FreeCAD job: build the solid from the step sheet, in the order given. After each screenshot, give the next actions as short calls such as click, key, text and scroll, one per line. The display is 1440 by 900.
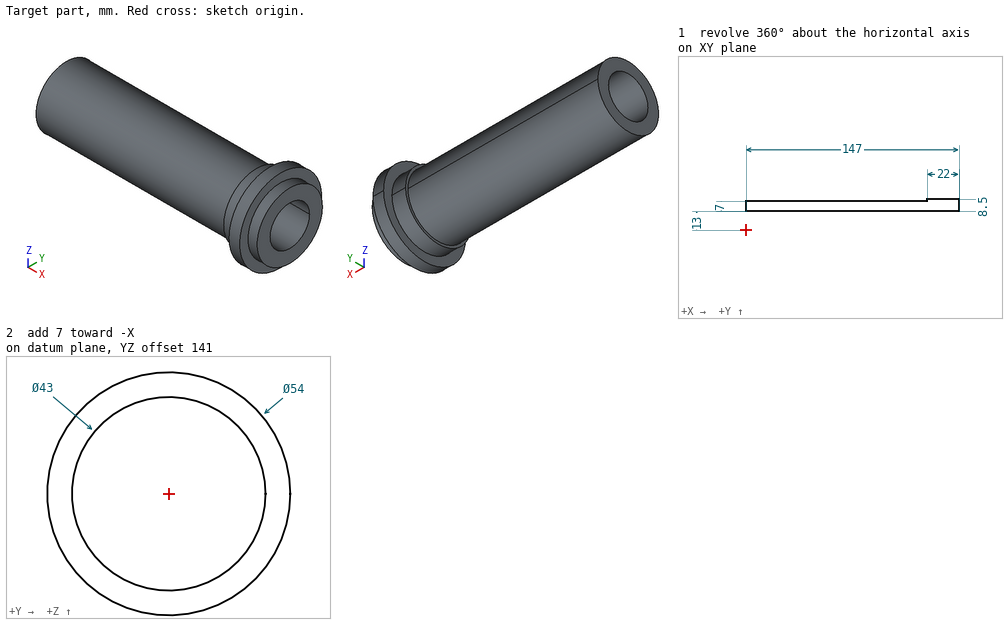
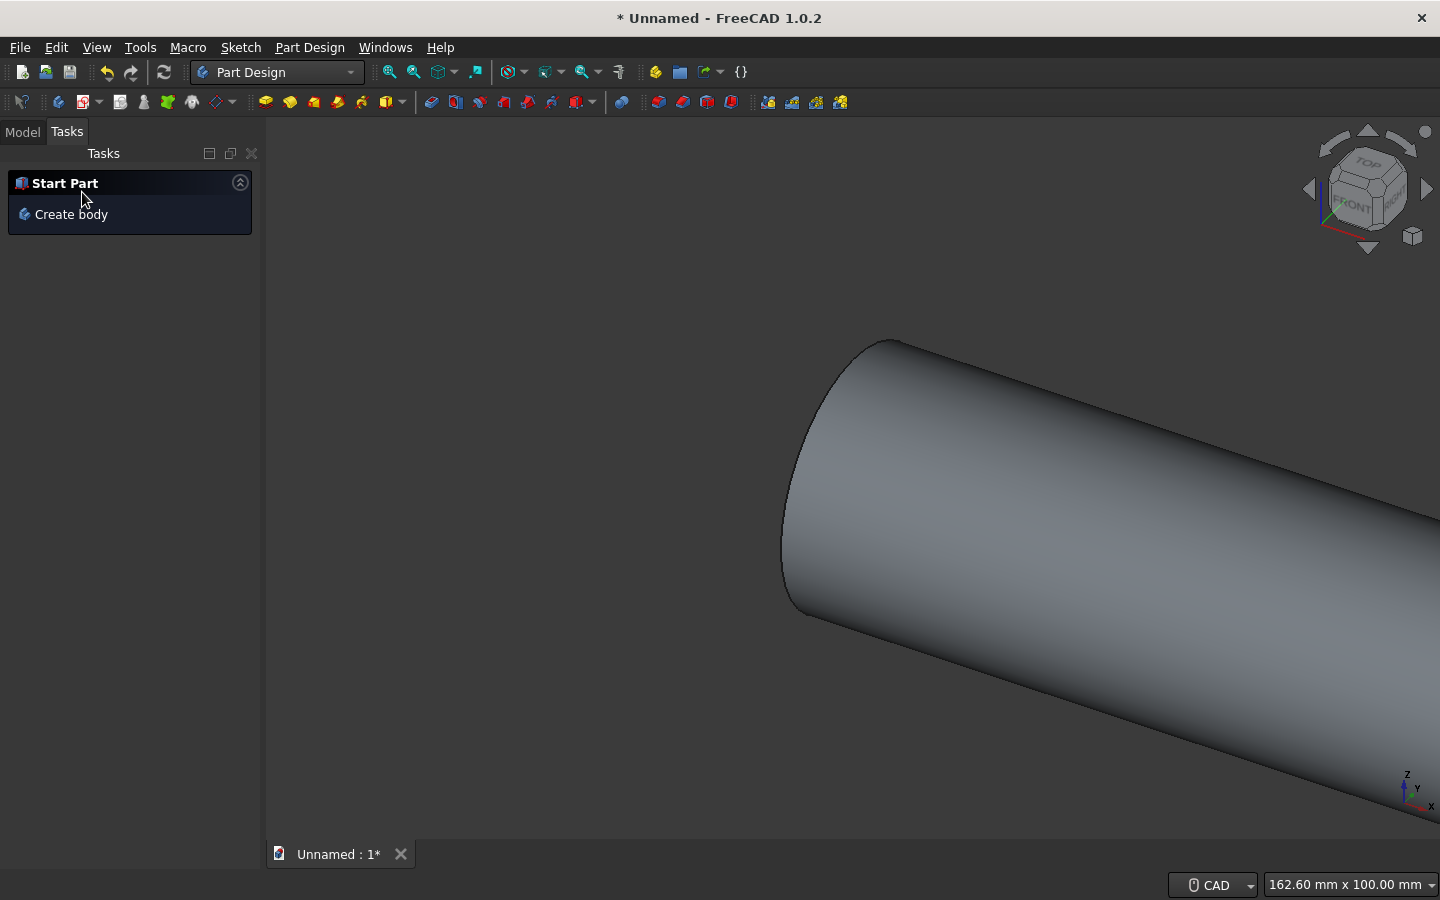
click(390, 72)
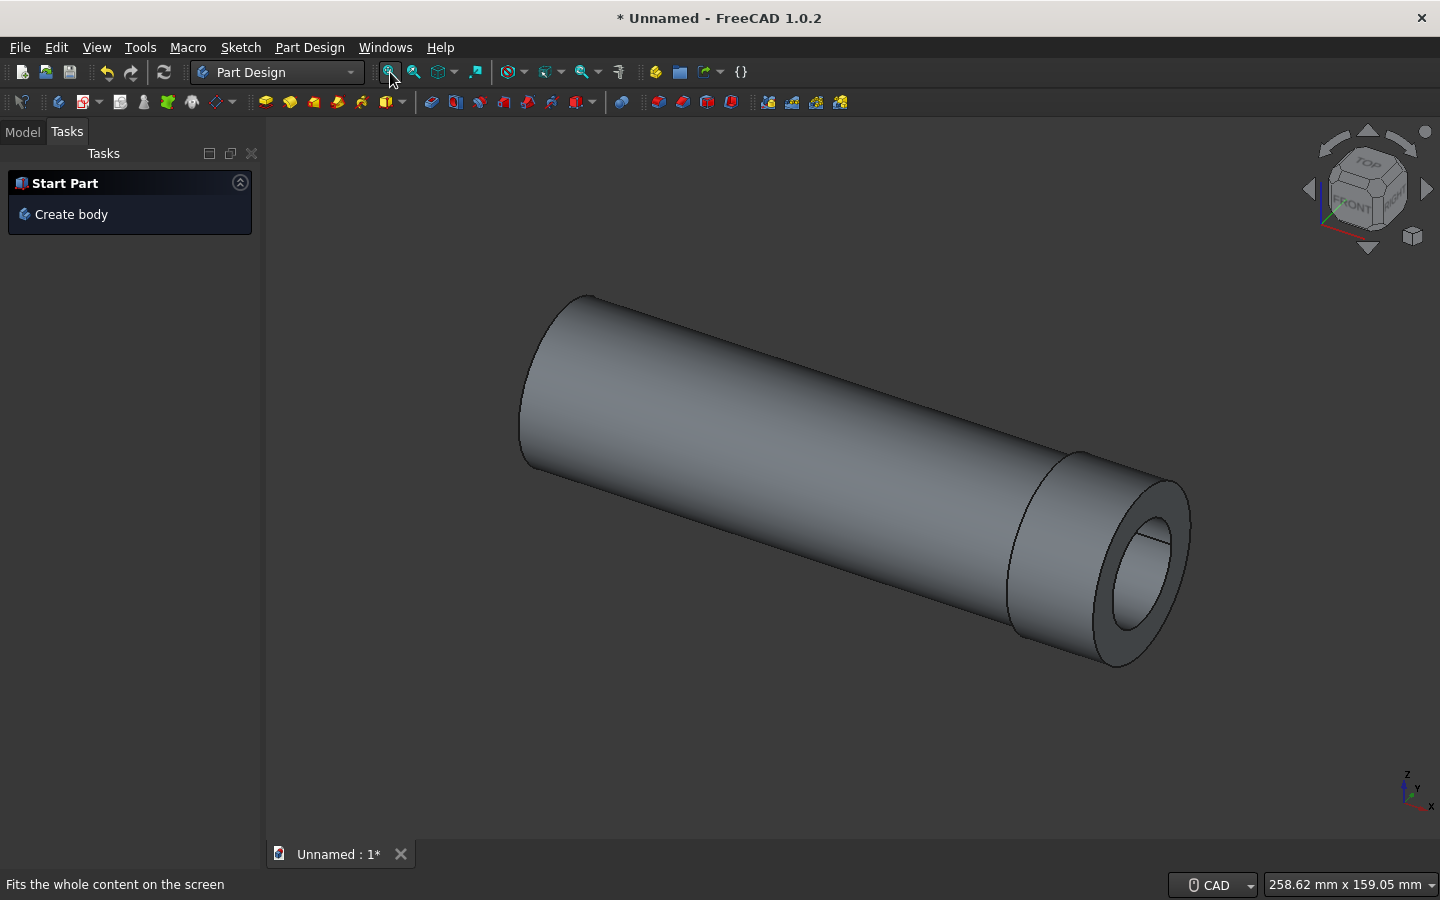
click(23, 131)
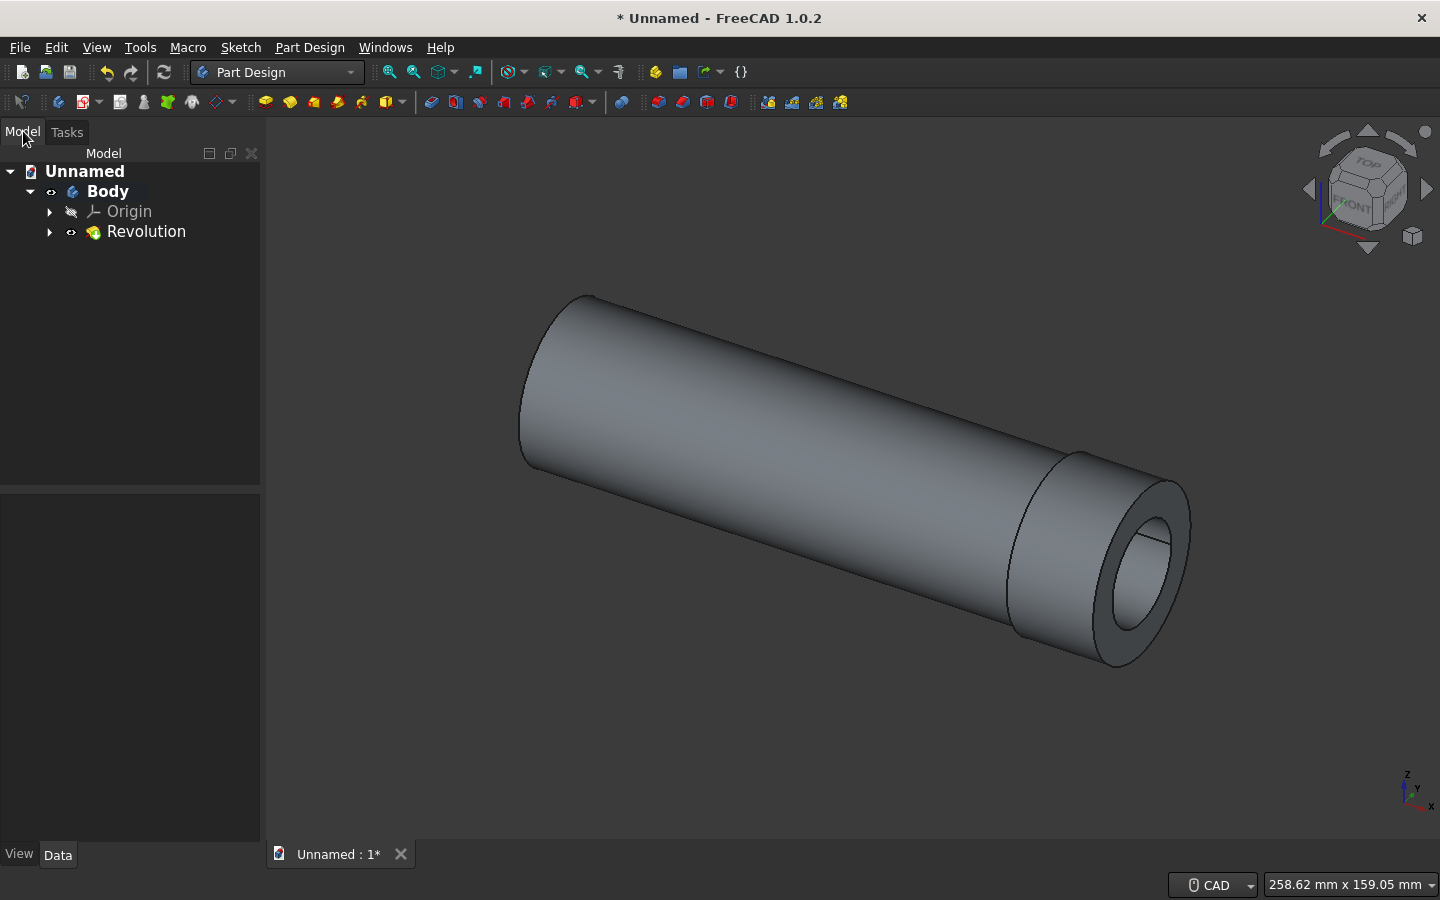
click(50, 212)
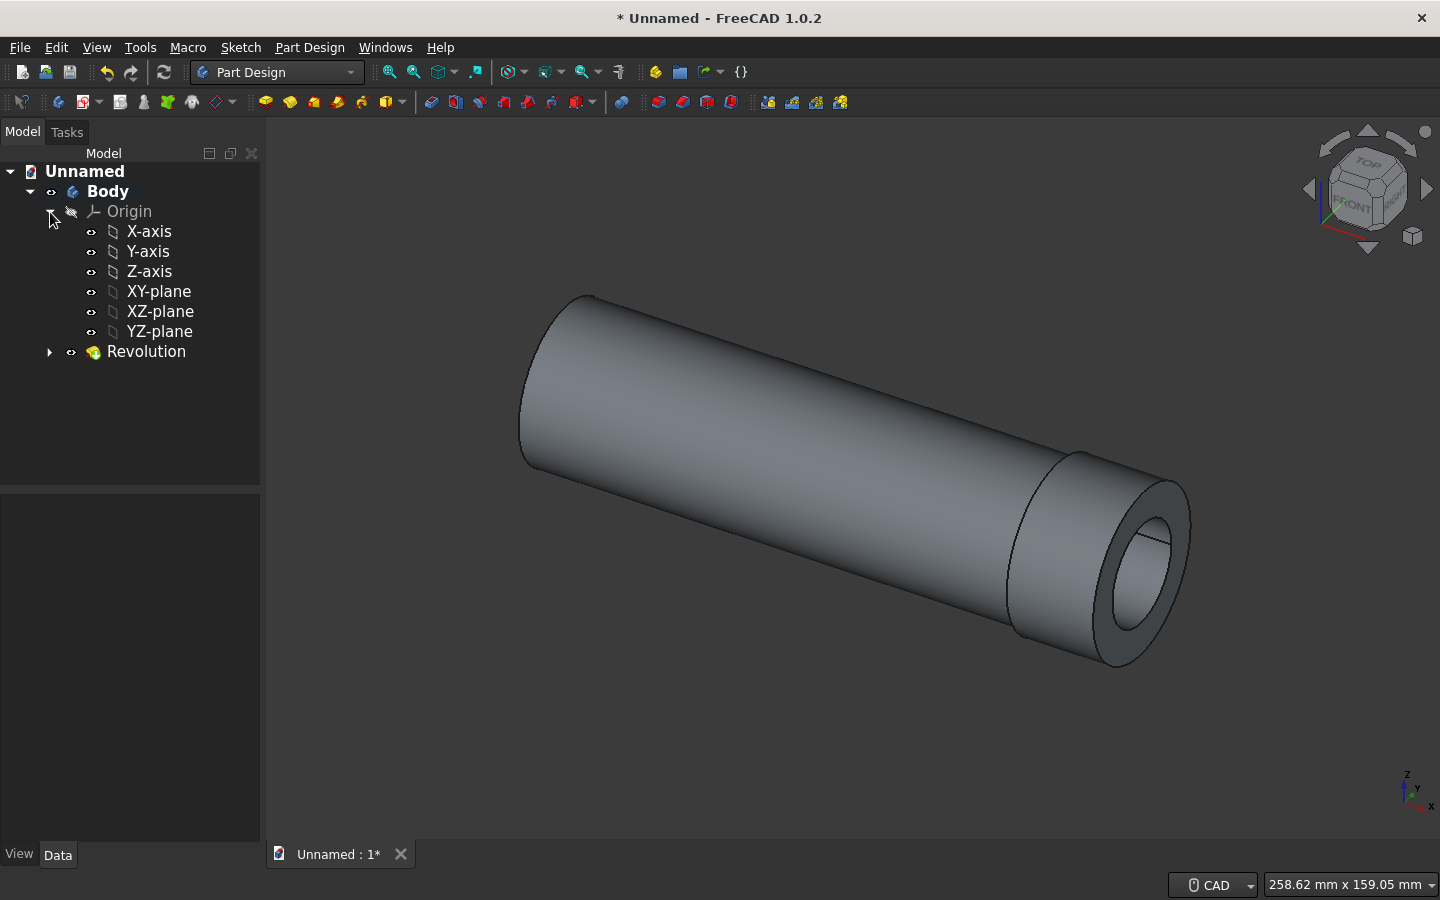
click(136, 332)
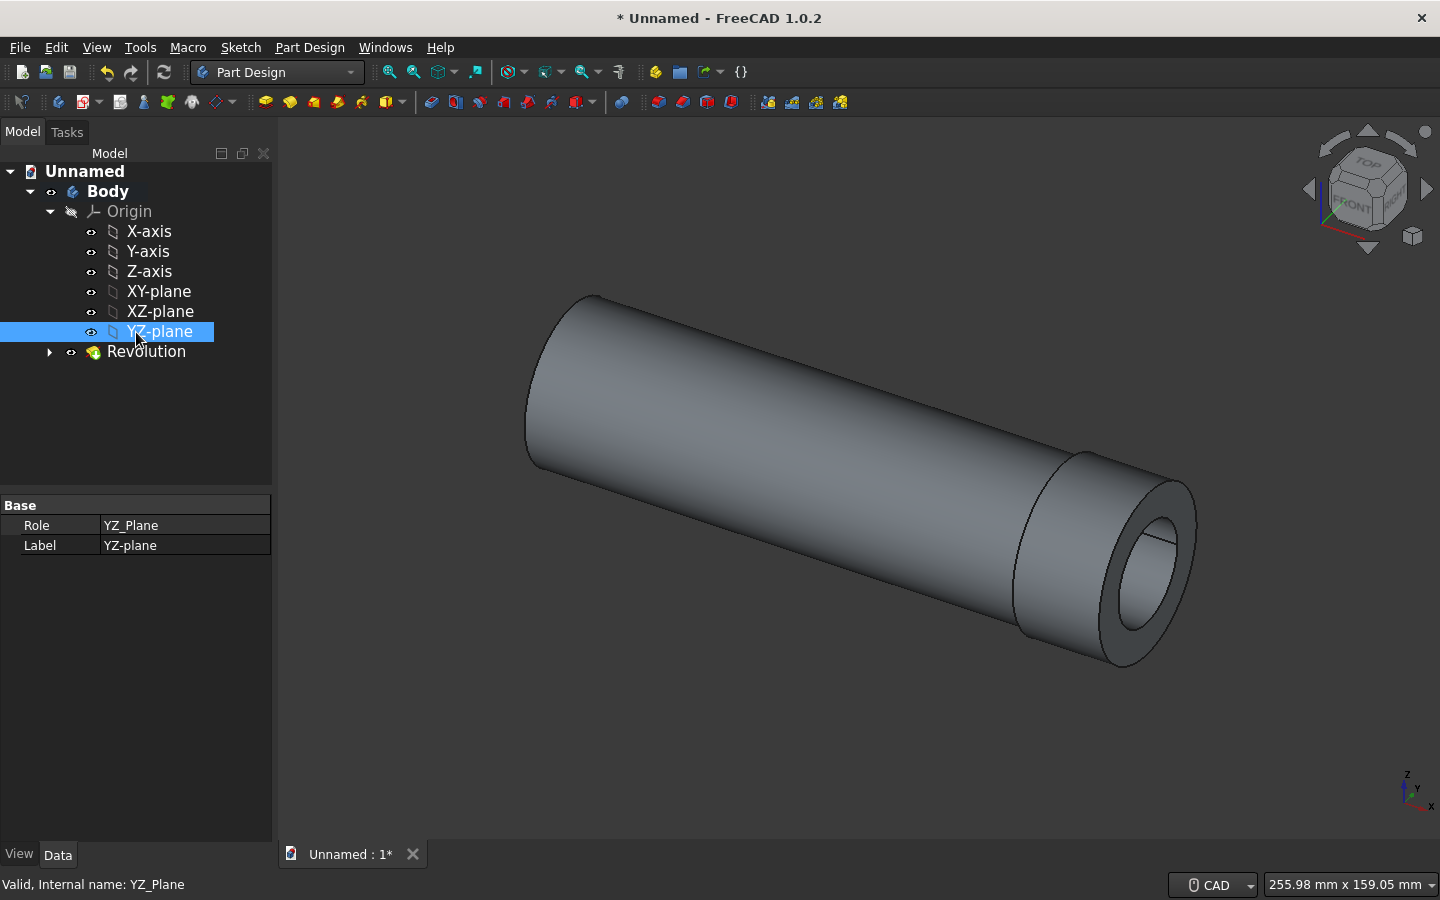
click(216, 102)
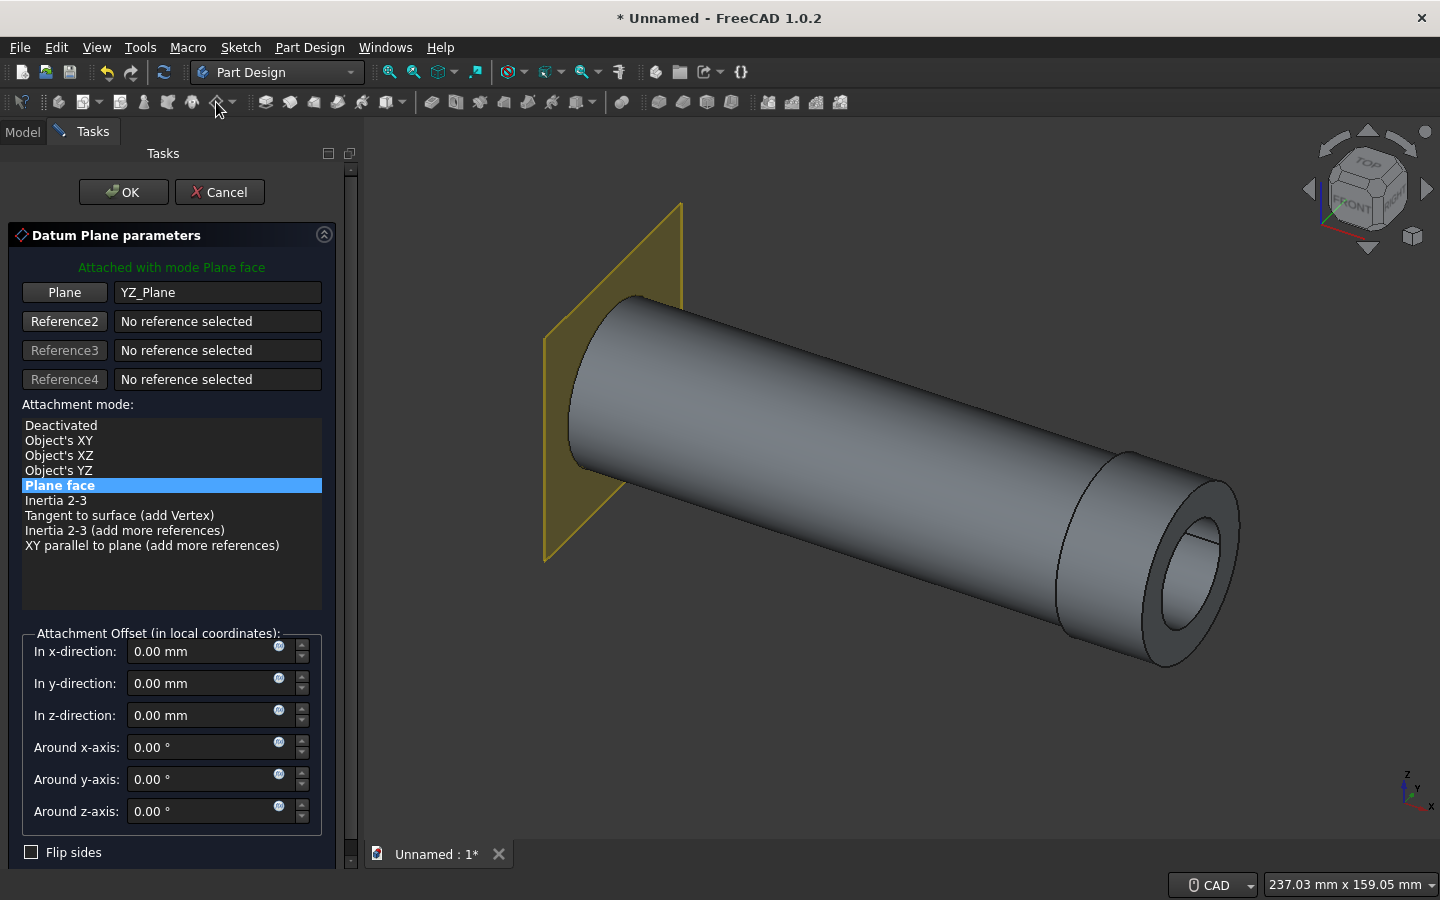
triple_click(210, 715)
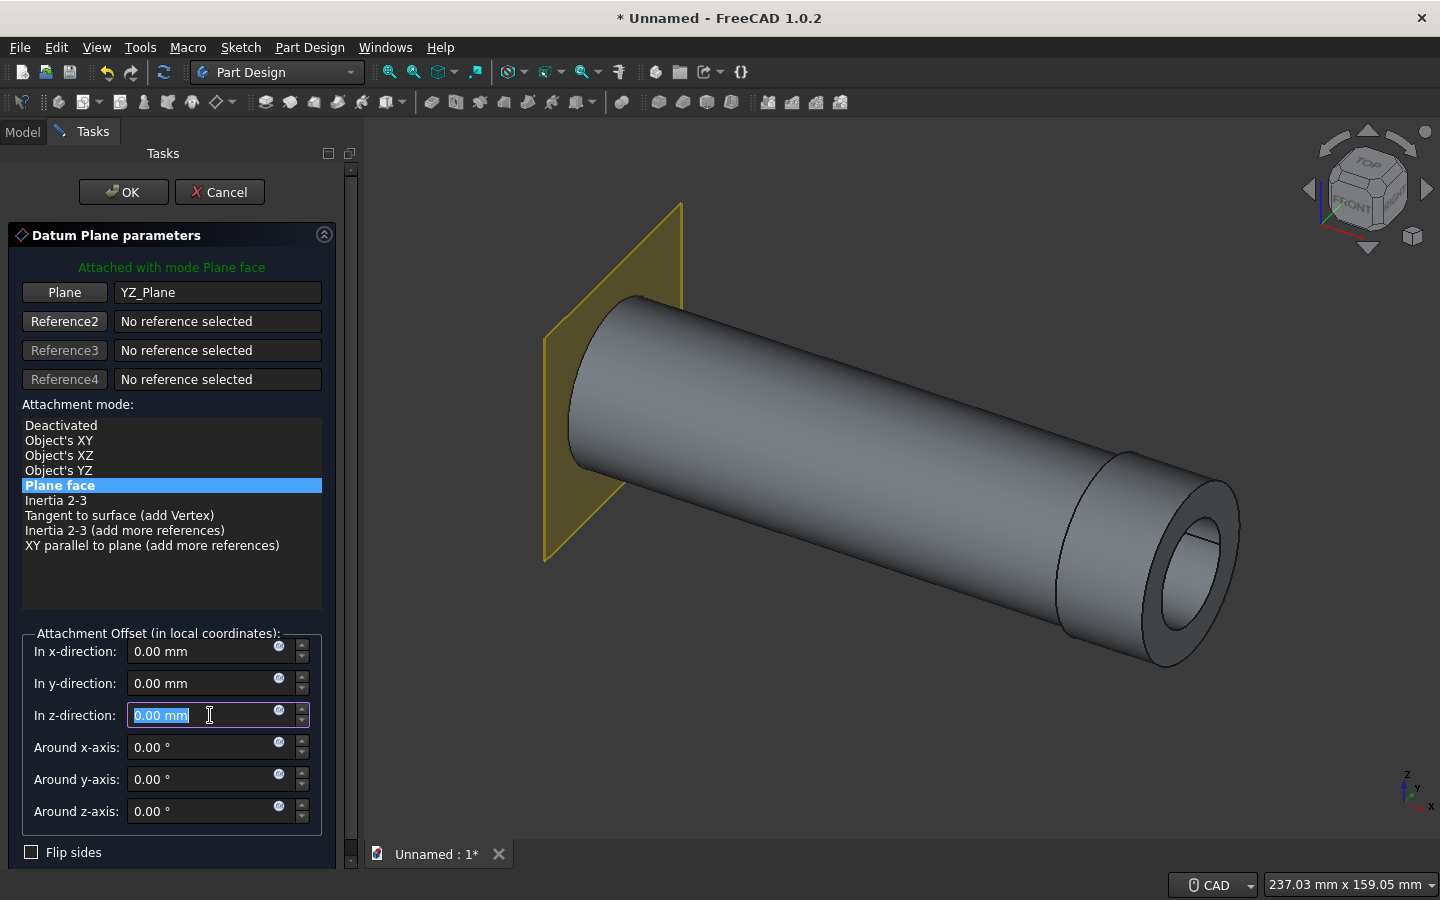
text(141)
key(Tab)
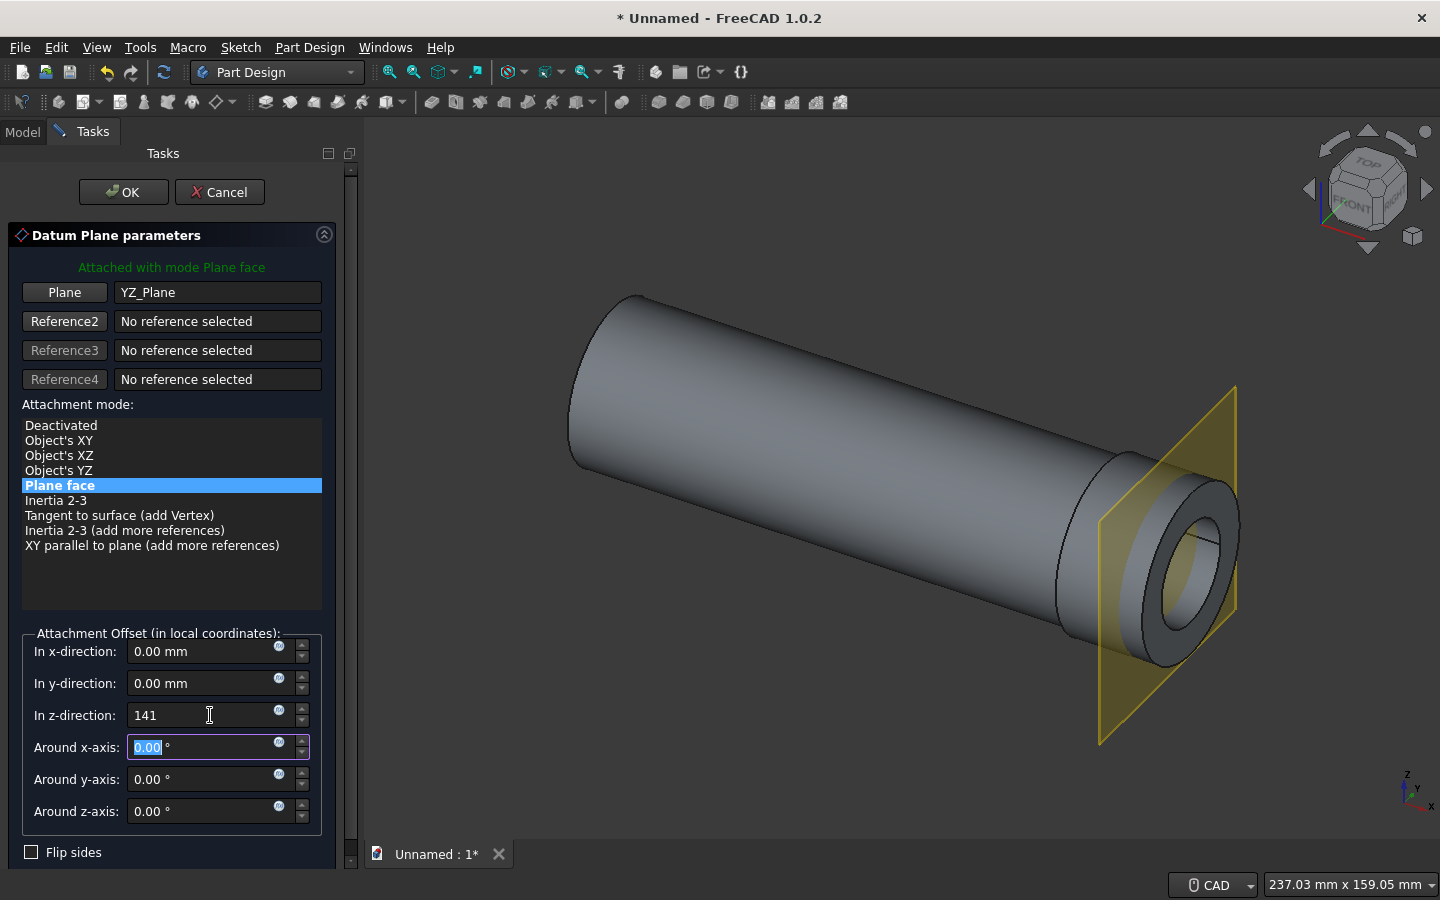
click(124, 192)